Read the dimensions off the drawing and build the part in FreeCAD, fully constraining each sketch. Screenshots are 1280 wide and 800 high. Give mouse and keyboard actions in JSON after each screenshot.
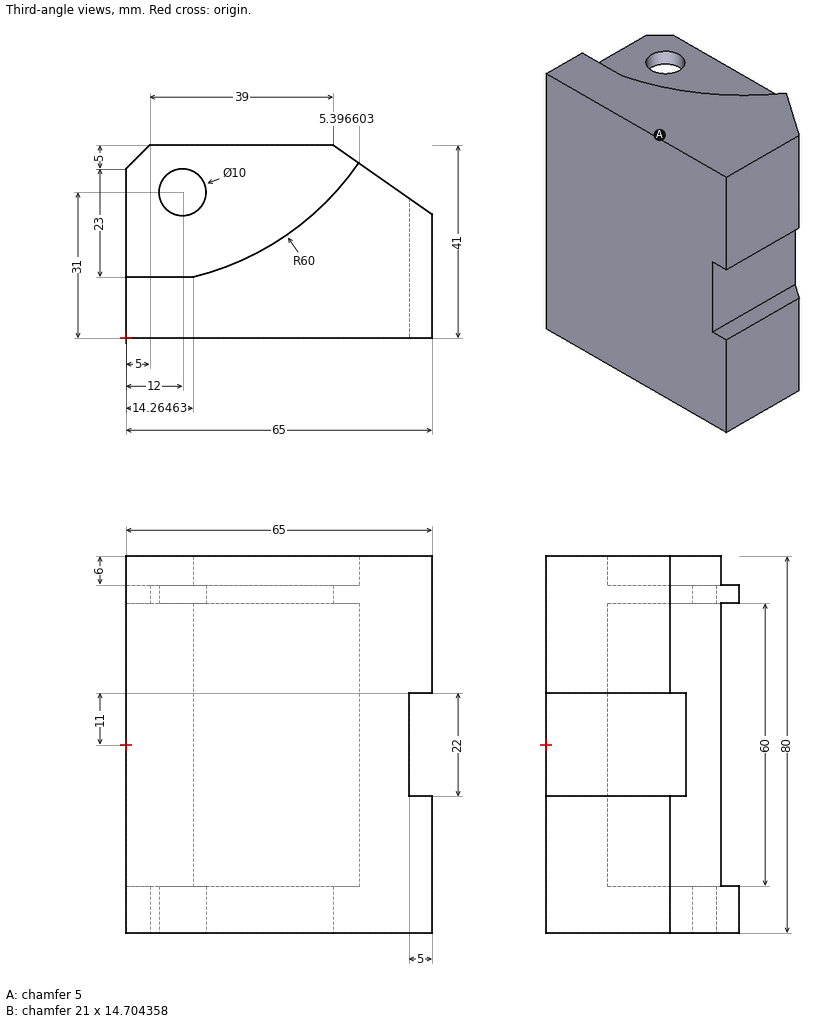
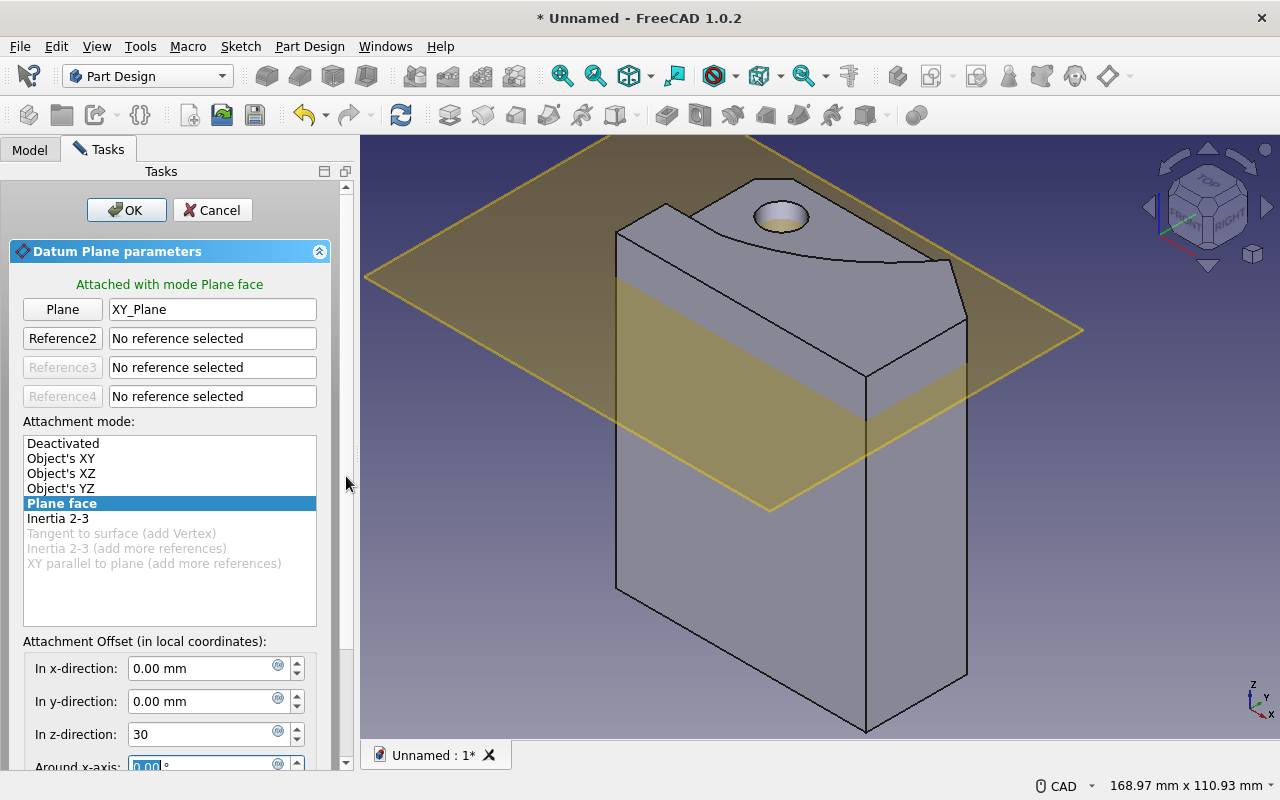
{"action": "left_click", "coordinate": [127, 210]}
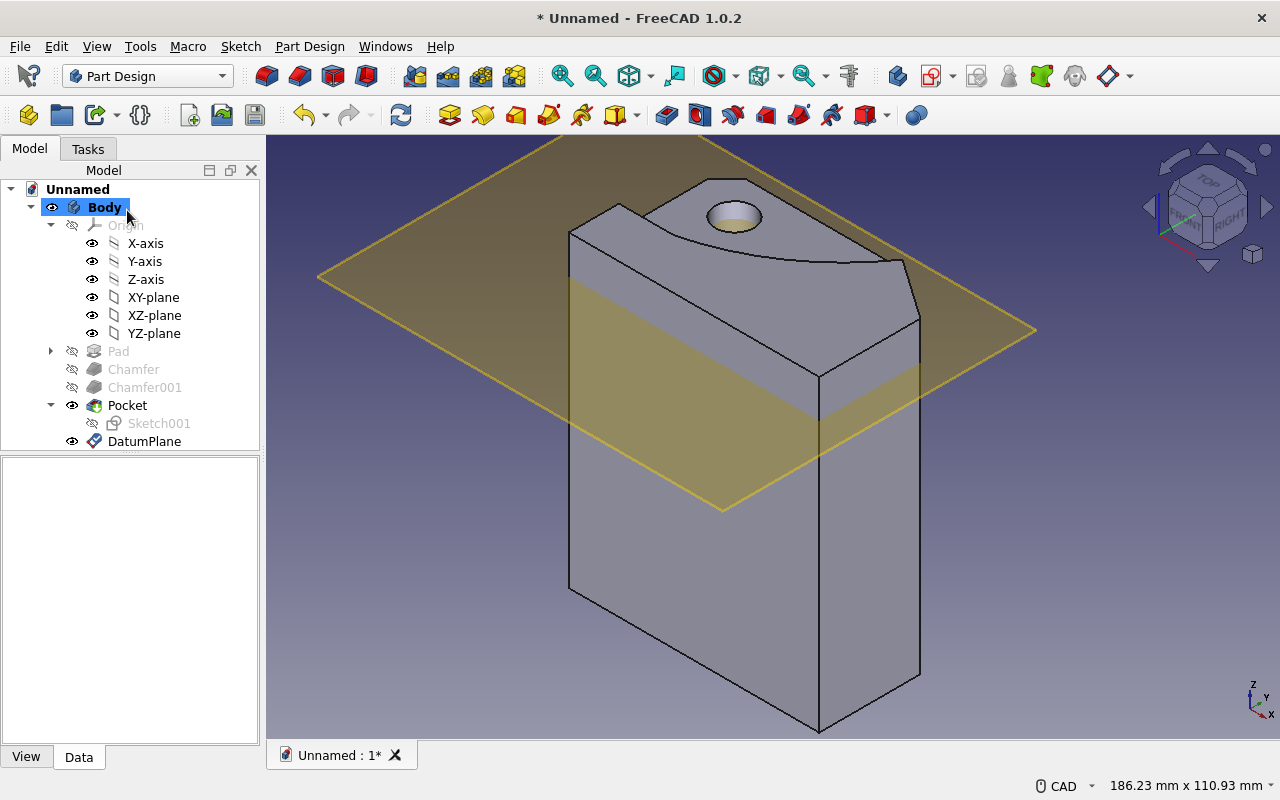
{"action": "left_click", "coordinate": [117, 441]}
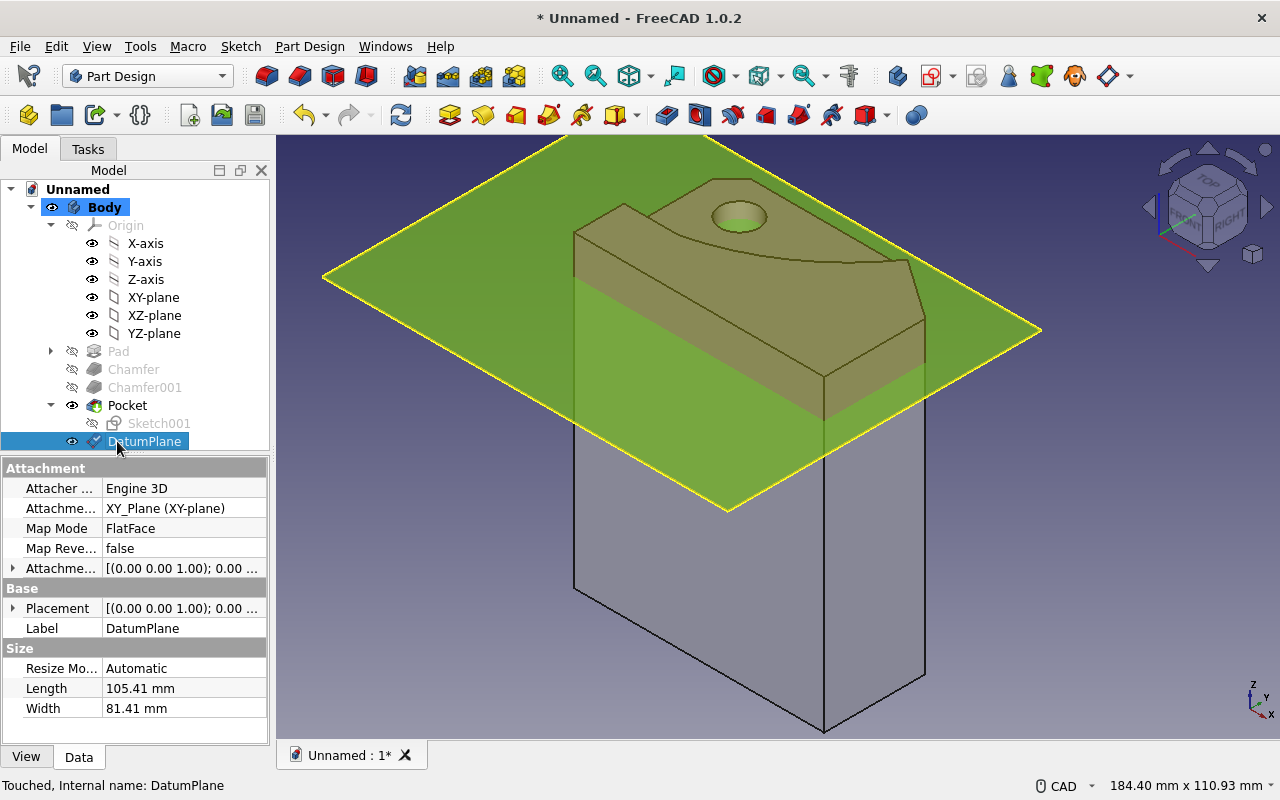
{"action": "left_click", "coordinate": [930, 76]}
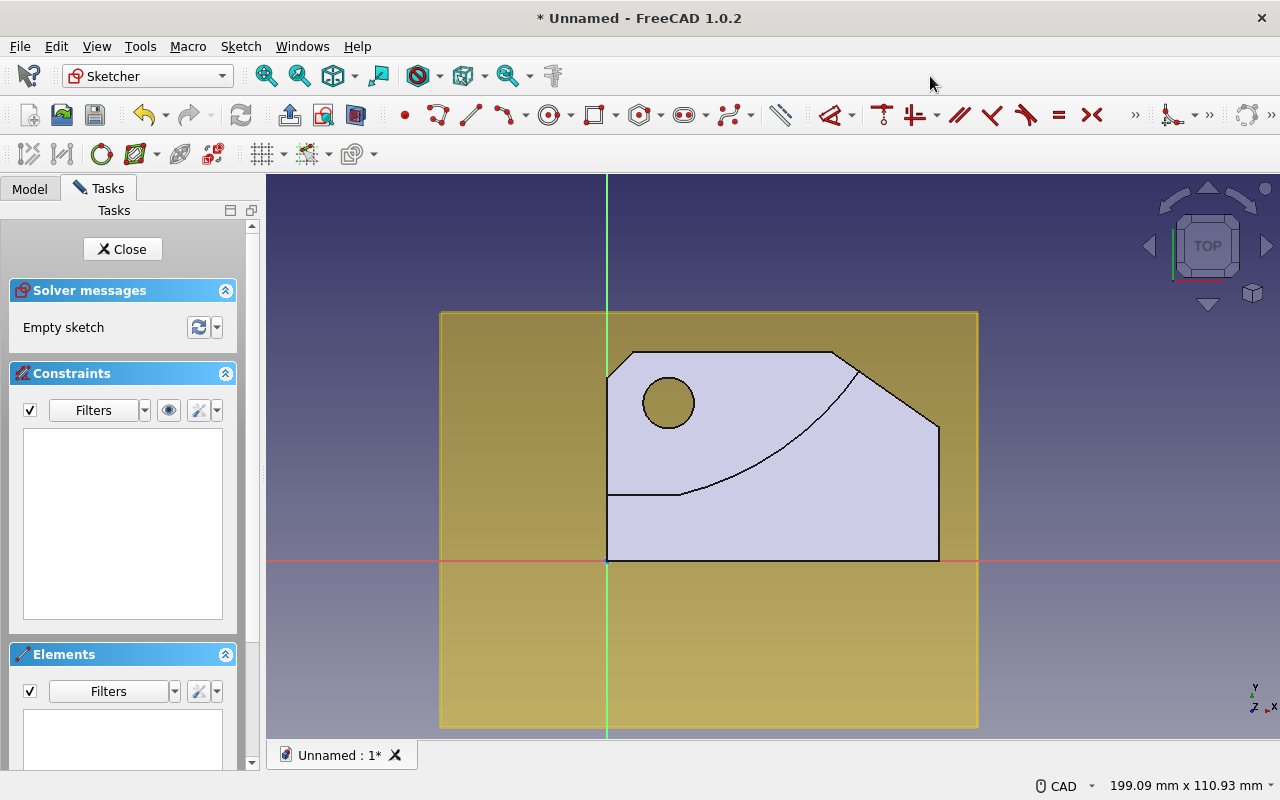
{"action": "key", "text": "q s"}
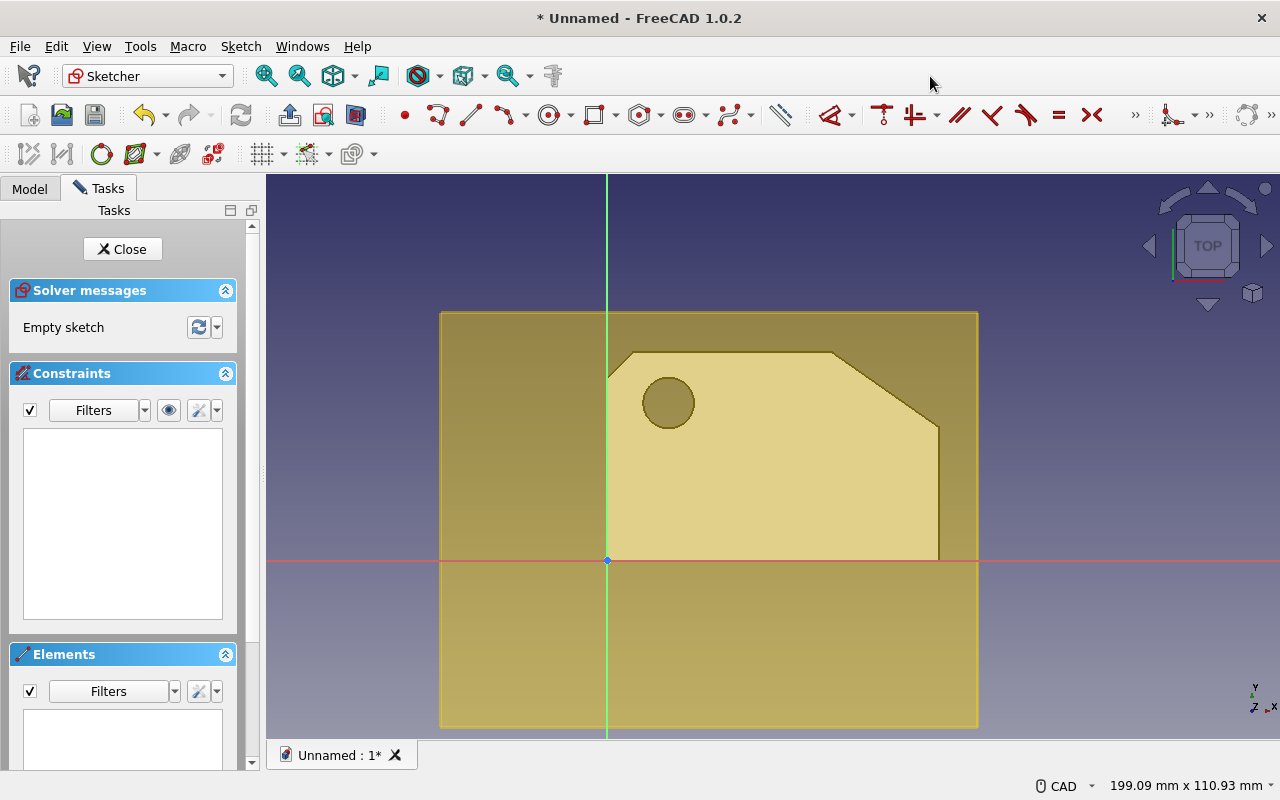
{"action": "scroll", "coordinate": [768, 456], "scroll_direction": "up", "scroll_amount": 3}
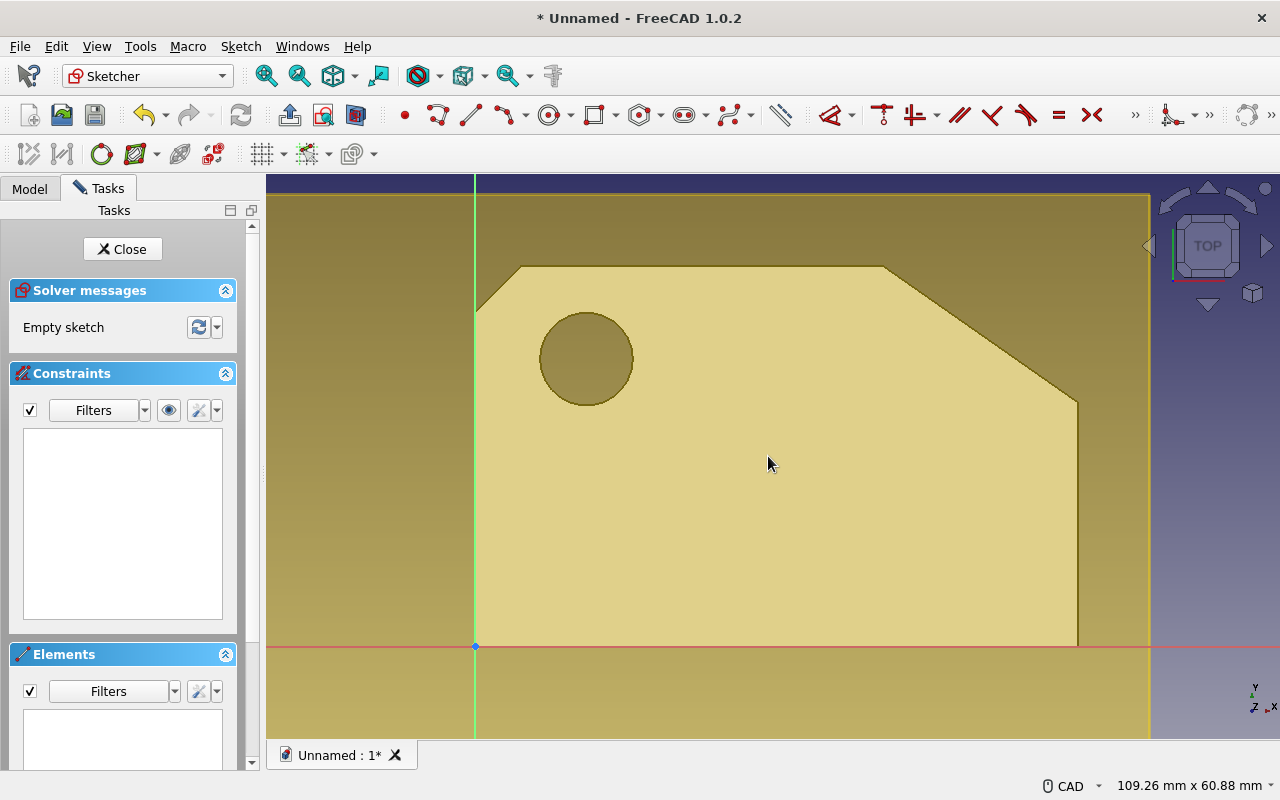
{"action": "left_click", "coordinate": [438, 116]}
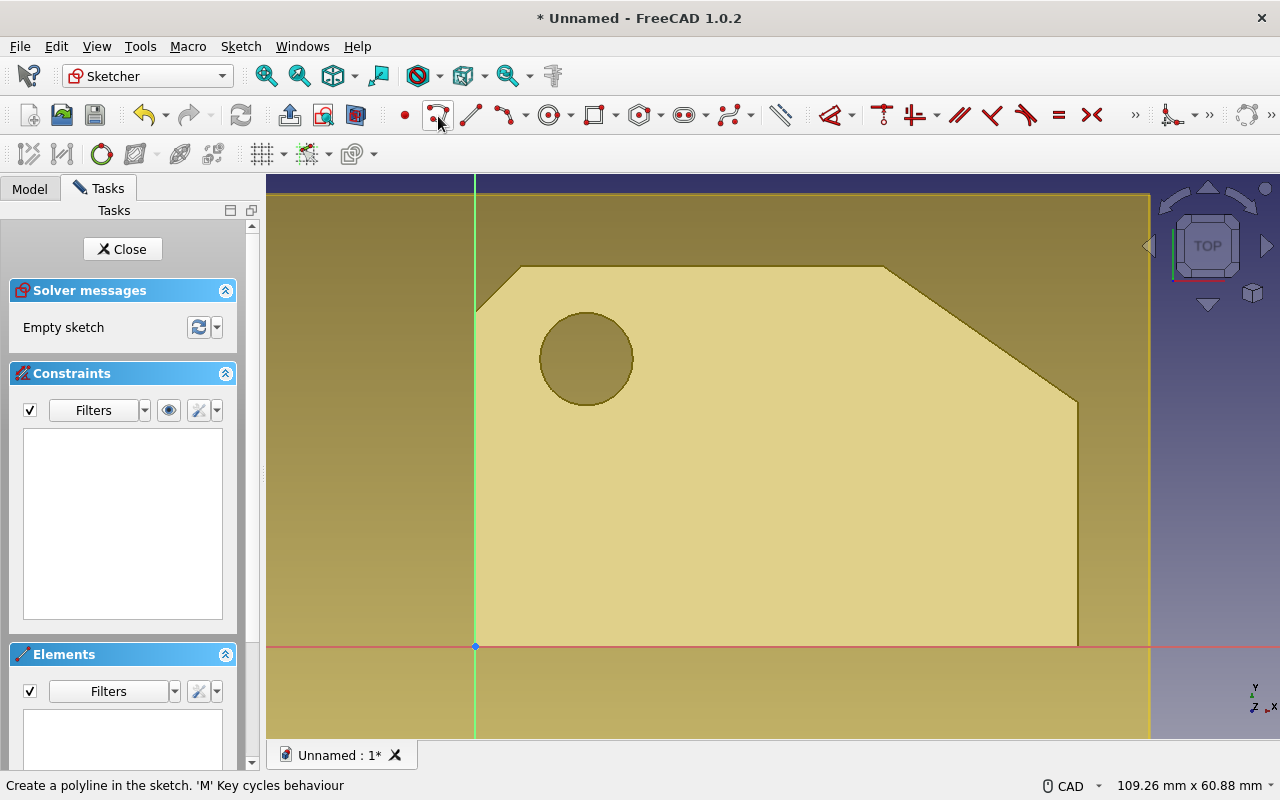
{"action": "left_click", "coordinate": [934, 301]}
{"action": "left_click", "coordinate": [883, 266]}
{"action": "left_click", "coordinate": [521, 266]}
{"action": "left_click", "coordinate": [475, 313]}
{"action": "left_click", "coordinate": [484, 526]}
{"action": "left_click", "coordinate": [607, 526]}
{"action": "right_click", "coordinate": [607, 526]}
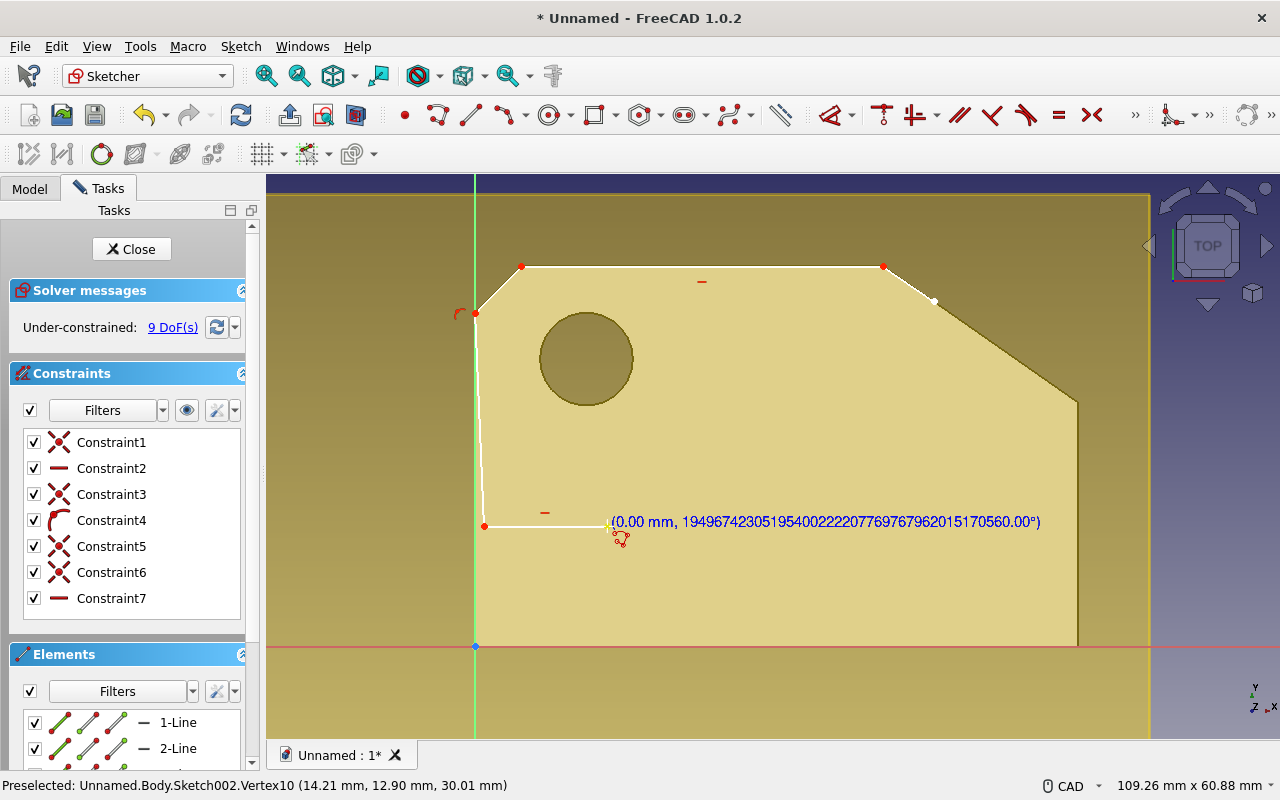
{"action": "left_click", "coordinate": [504, 116]}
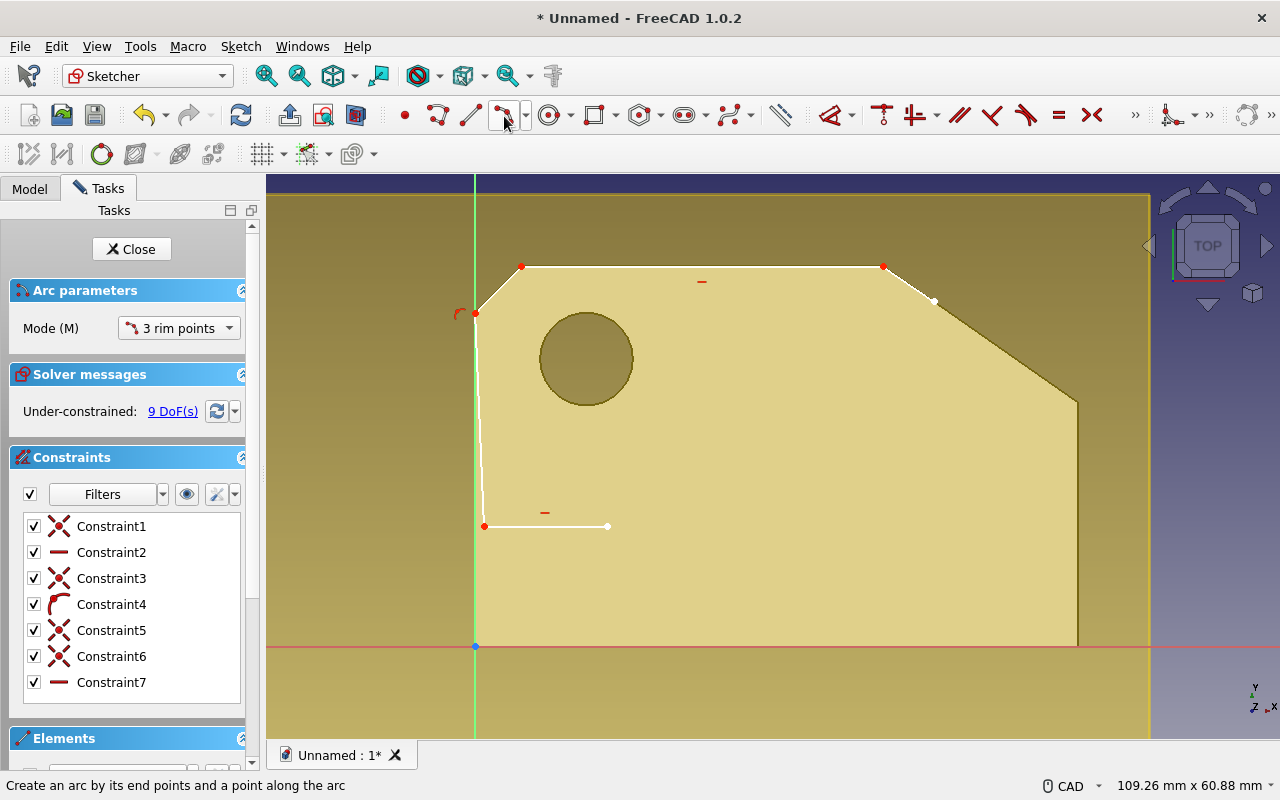
{"action": "left_click", "coordinate": [607, 527]}
{"action": "left_click", "coordinate": [934, 302]}
{"action": "left_click", "coordinate": [791, 444]}
{"action": "key", "text": "Escape"}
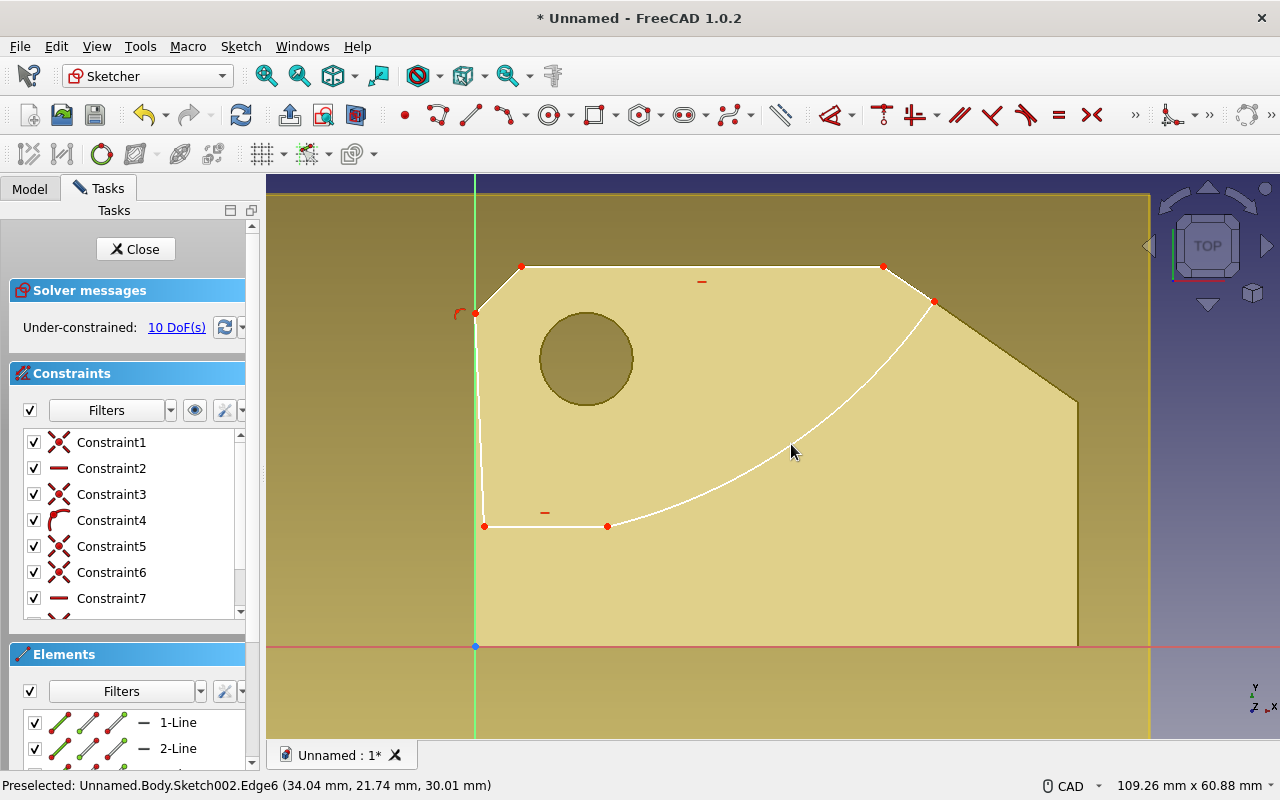
{"action": "left_click", "coordinate": [478, 378]}